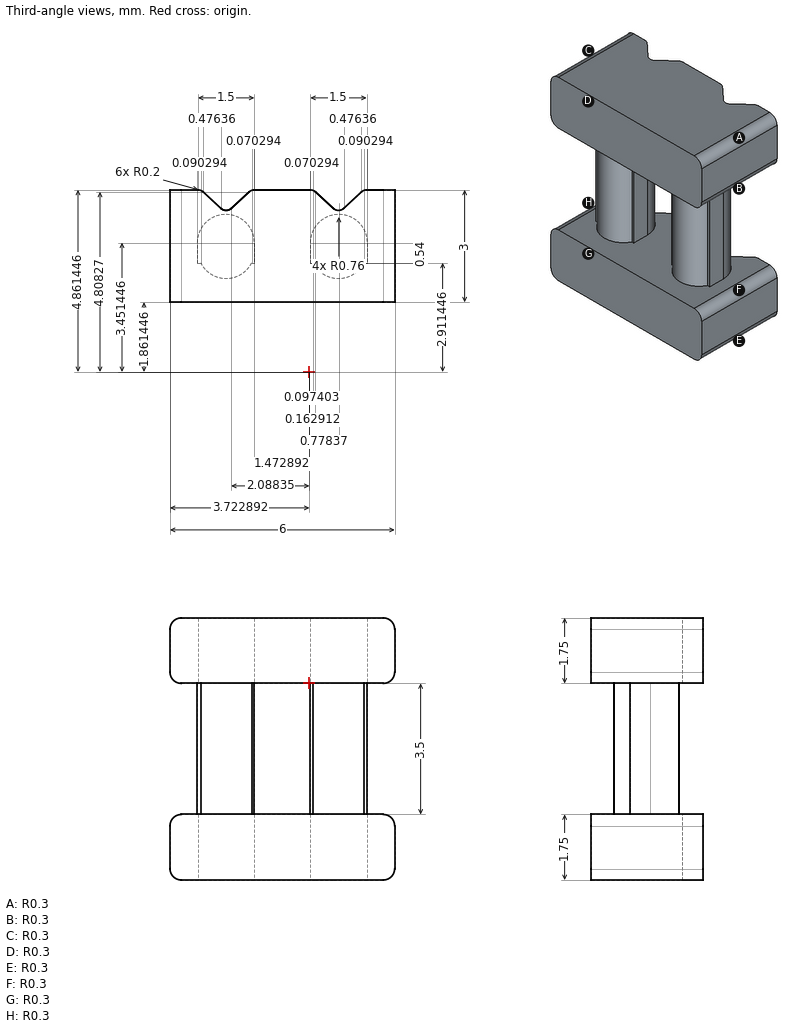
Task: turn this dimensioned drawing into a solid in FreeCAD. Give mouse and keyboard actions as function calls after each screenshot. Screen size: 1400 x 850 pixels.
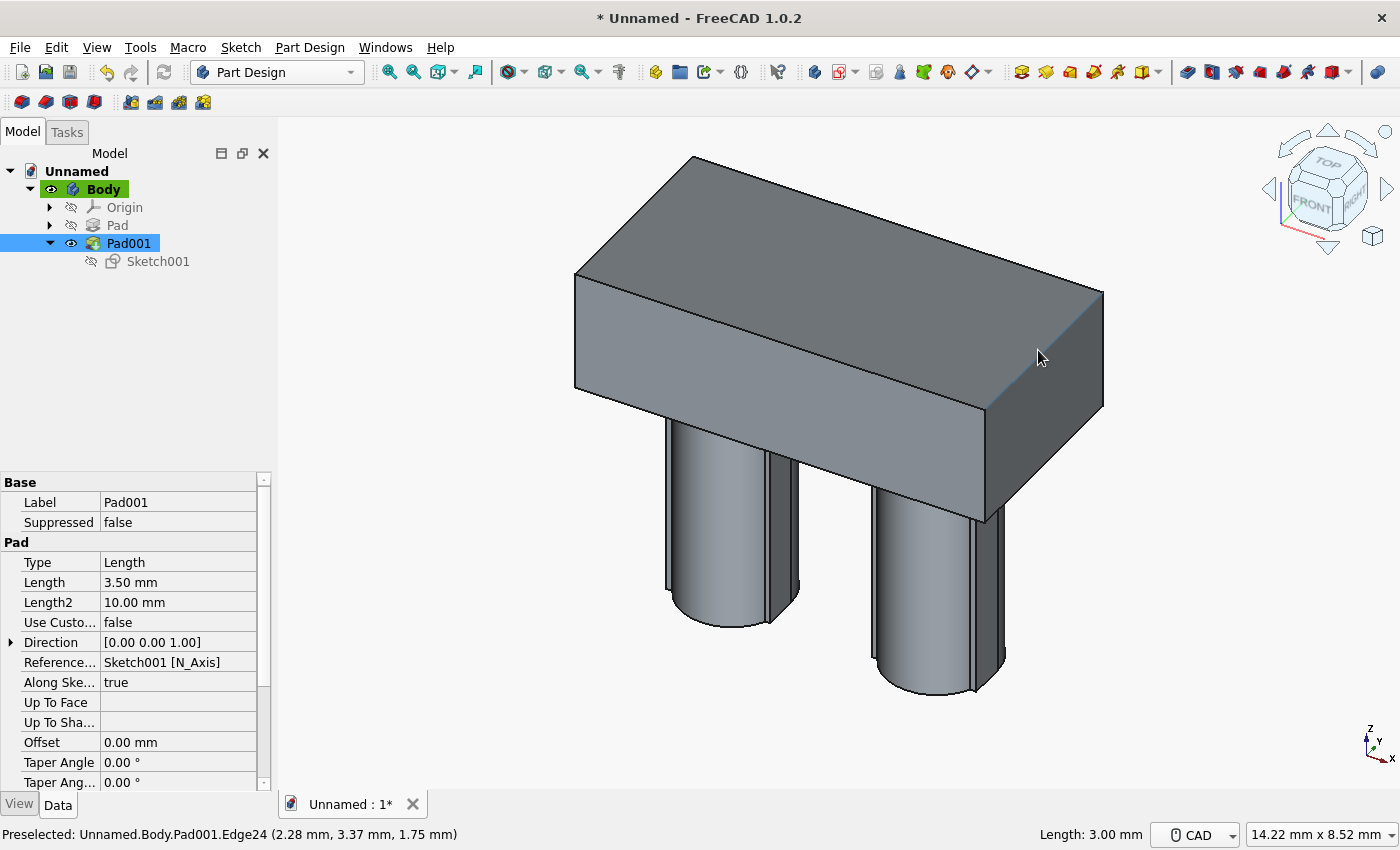
click(22, 102)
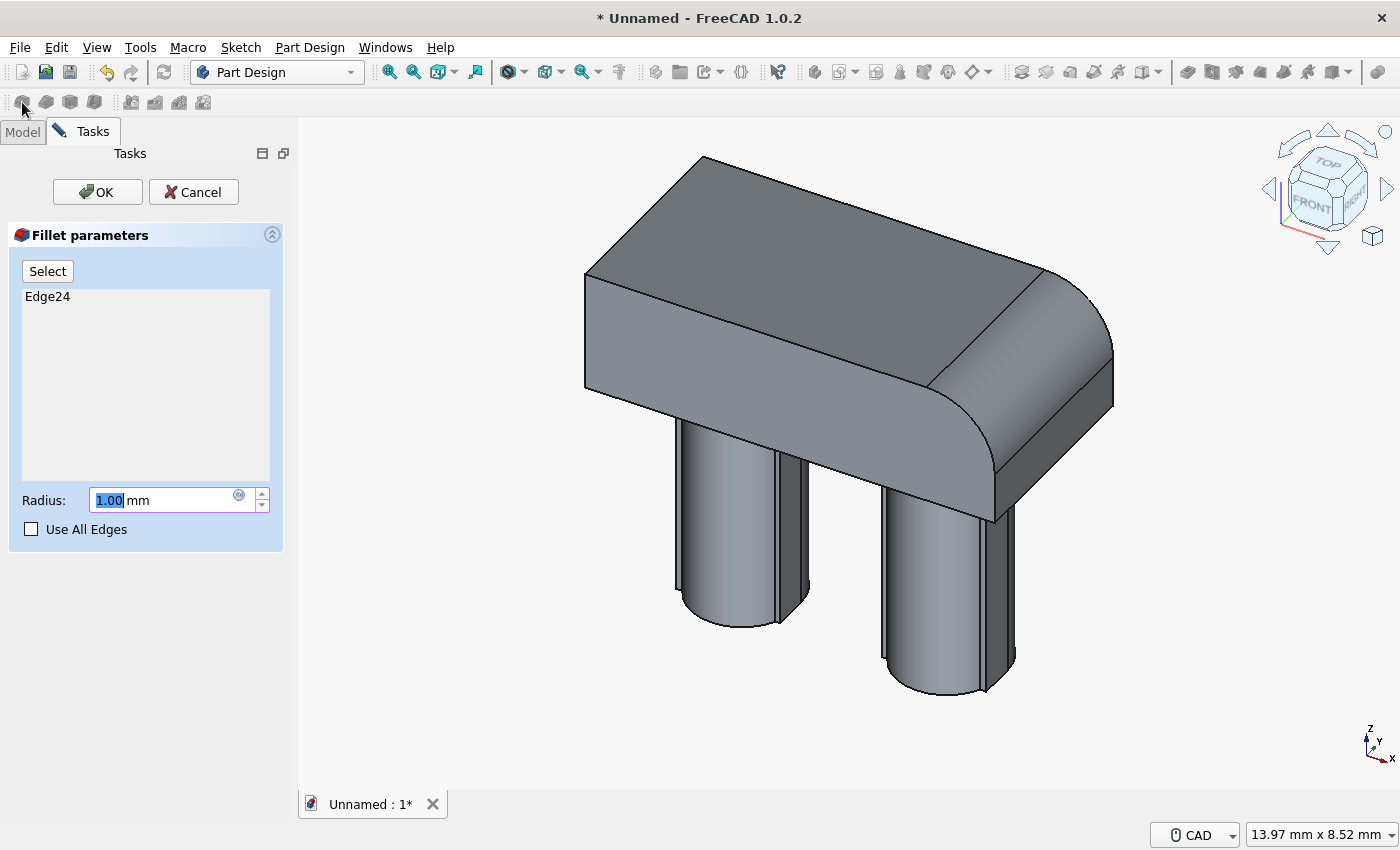
text(0.3)
key(Tab)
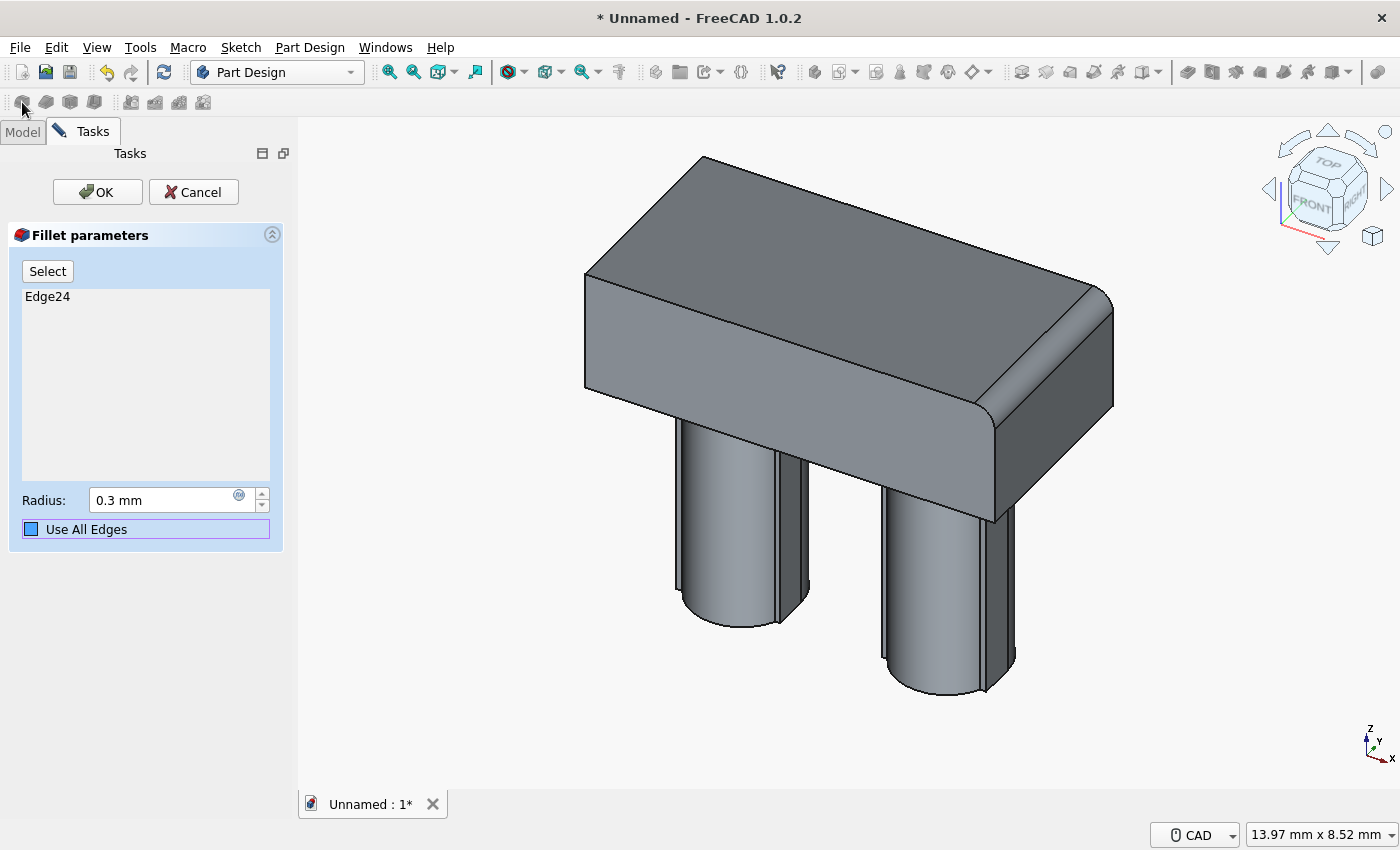
click(98, 192)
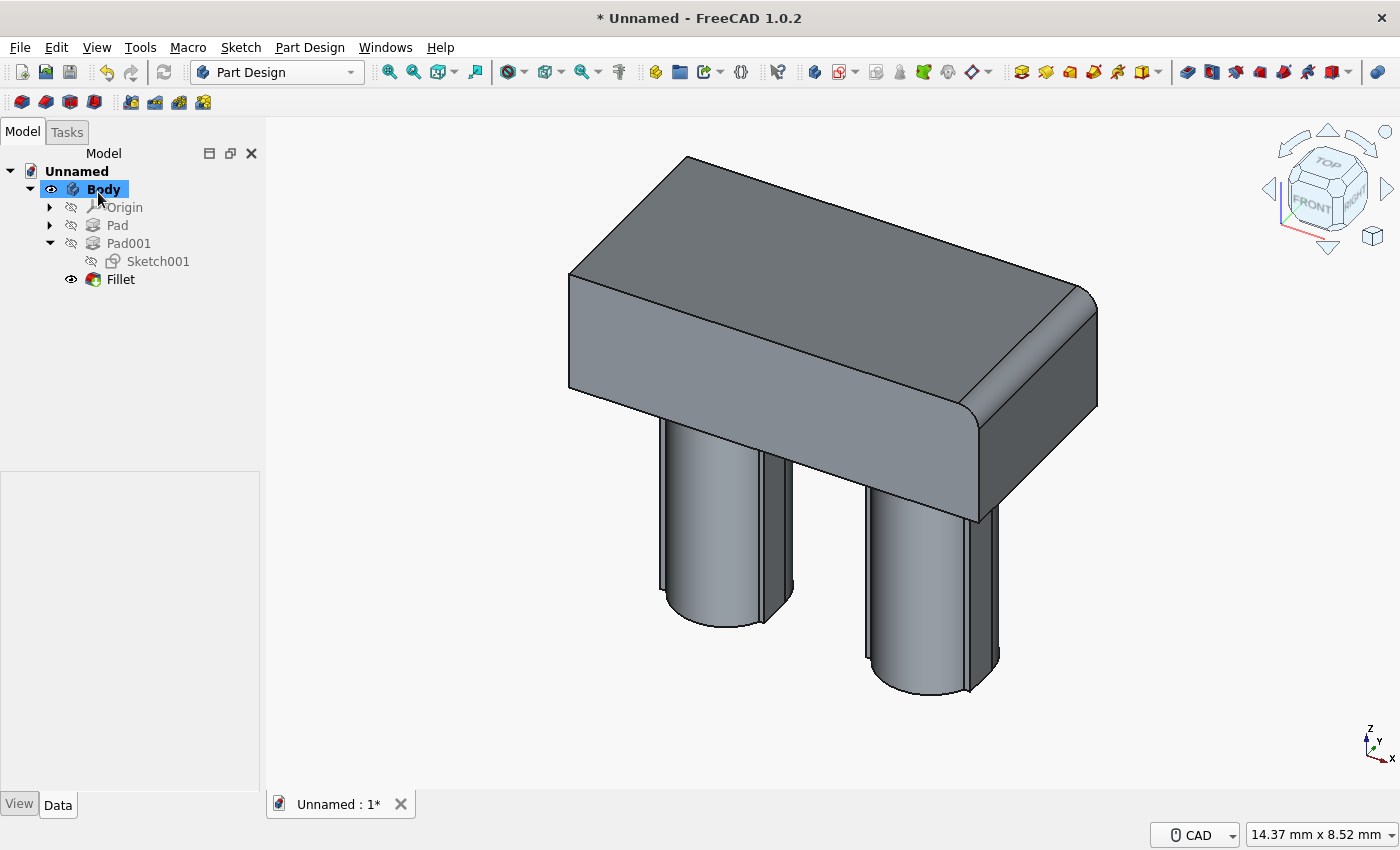
key(0)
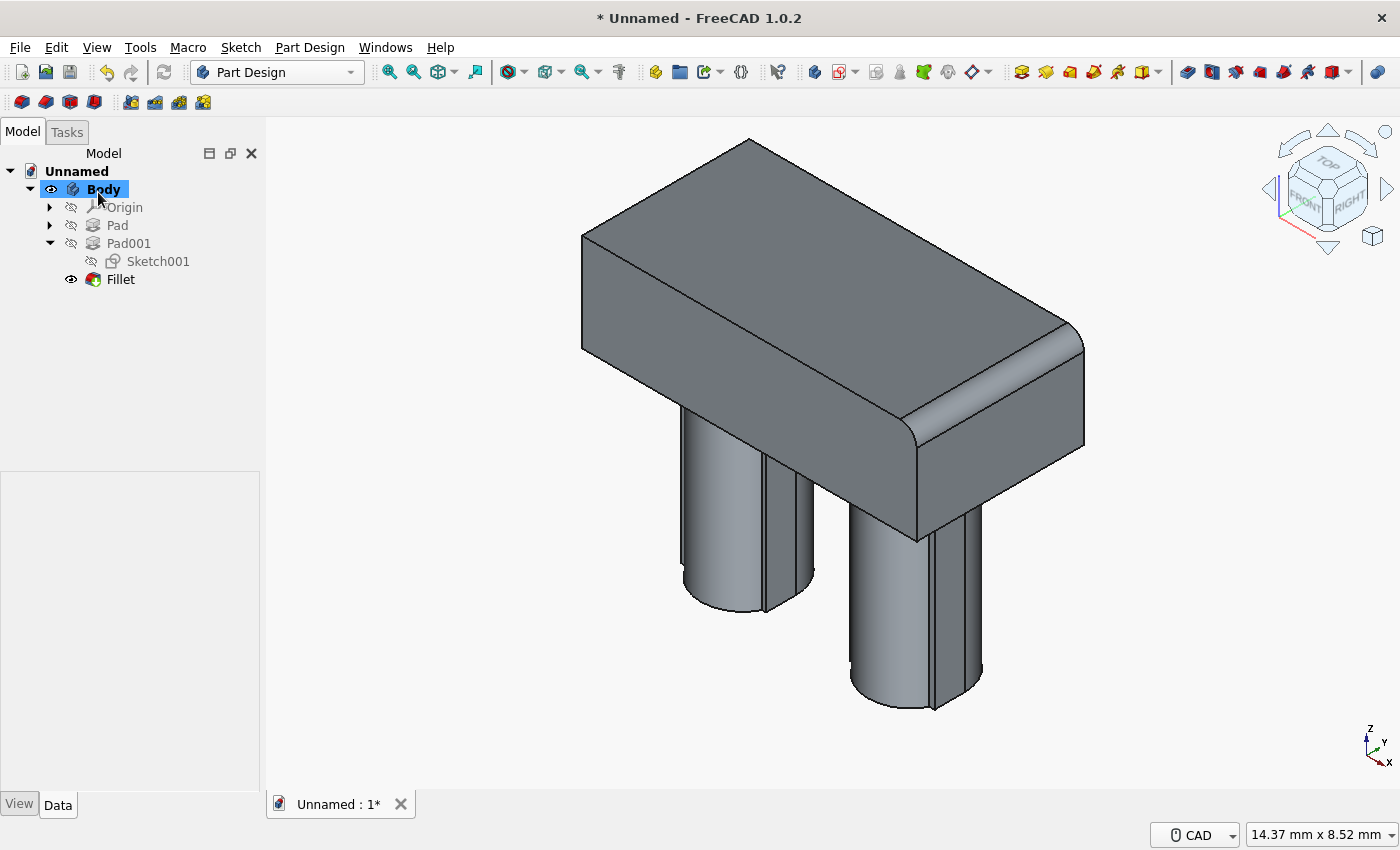
key(2)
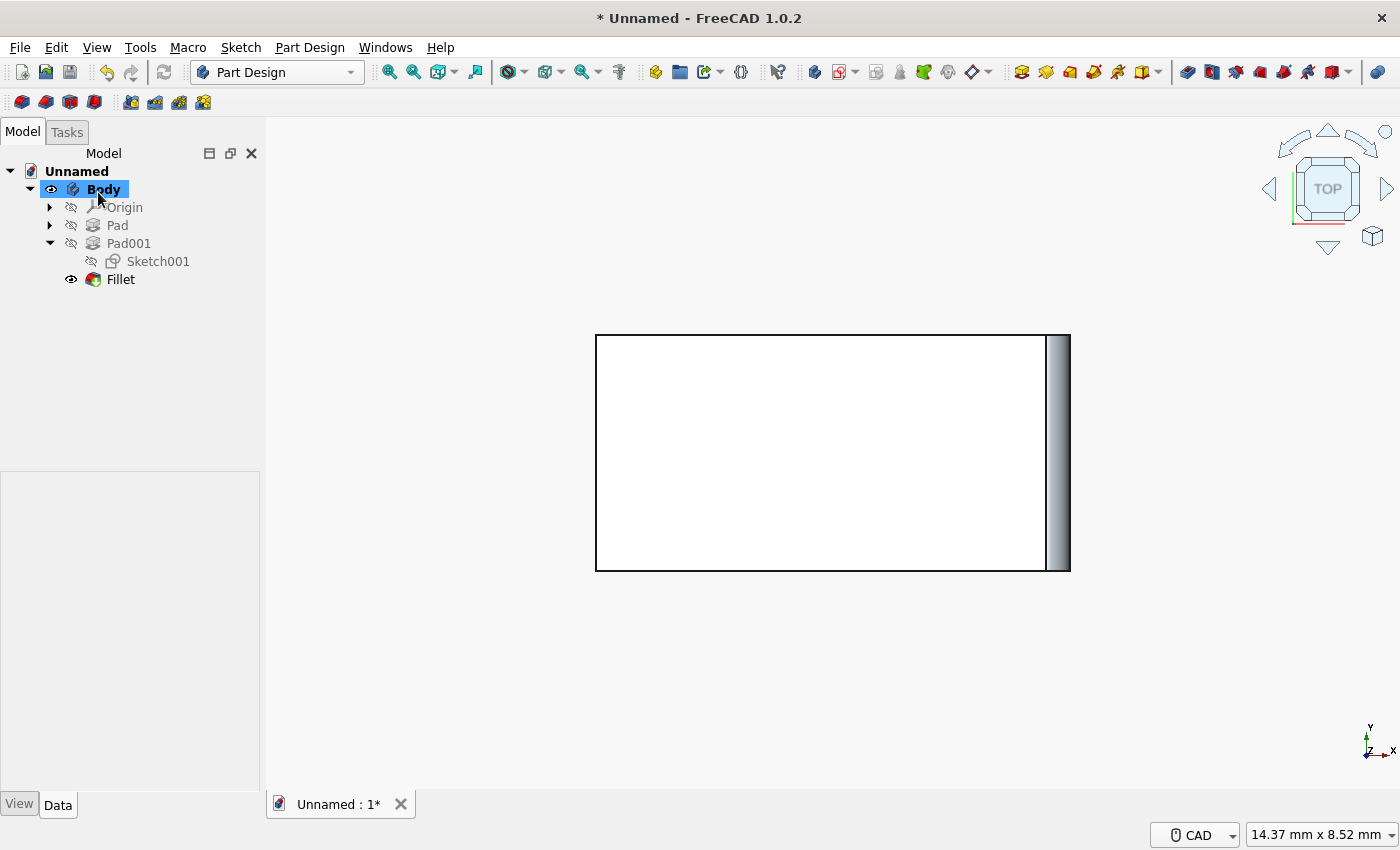
click(390, 72)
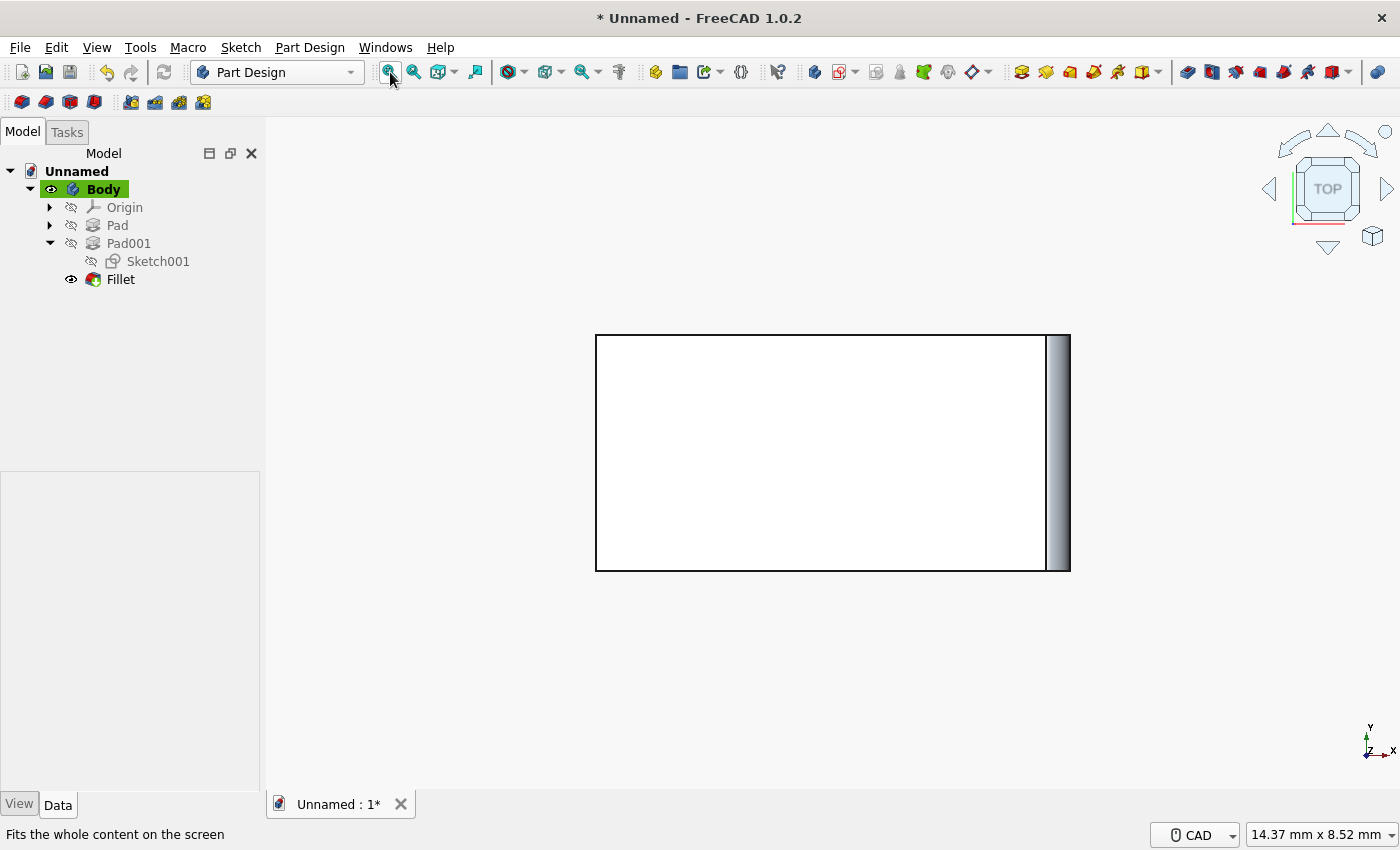
key(1)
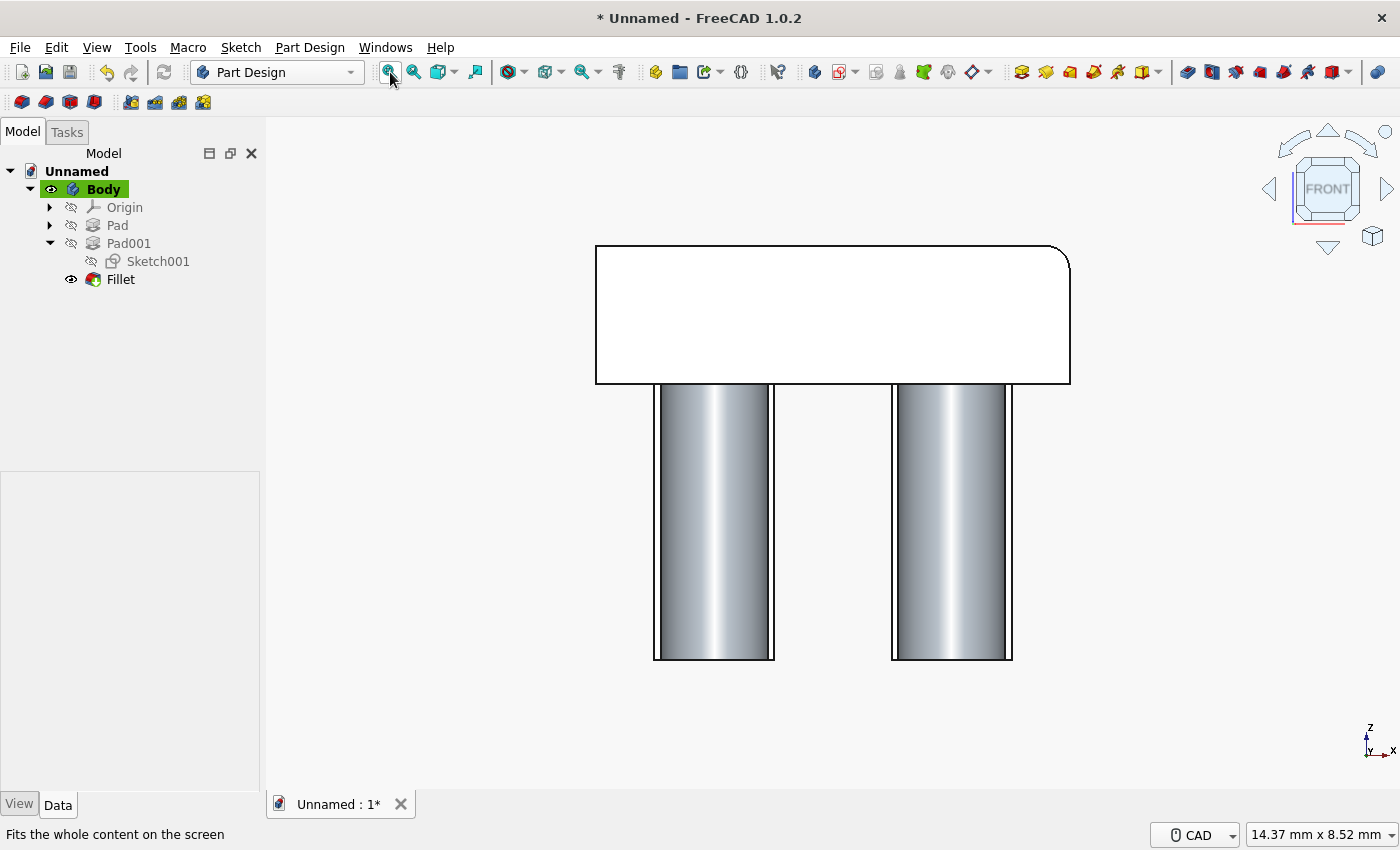
key(3)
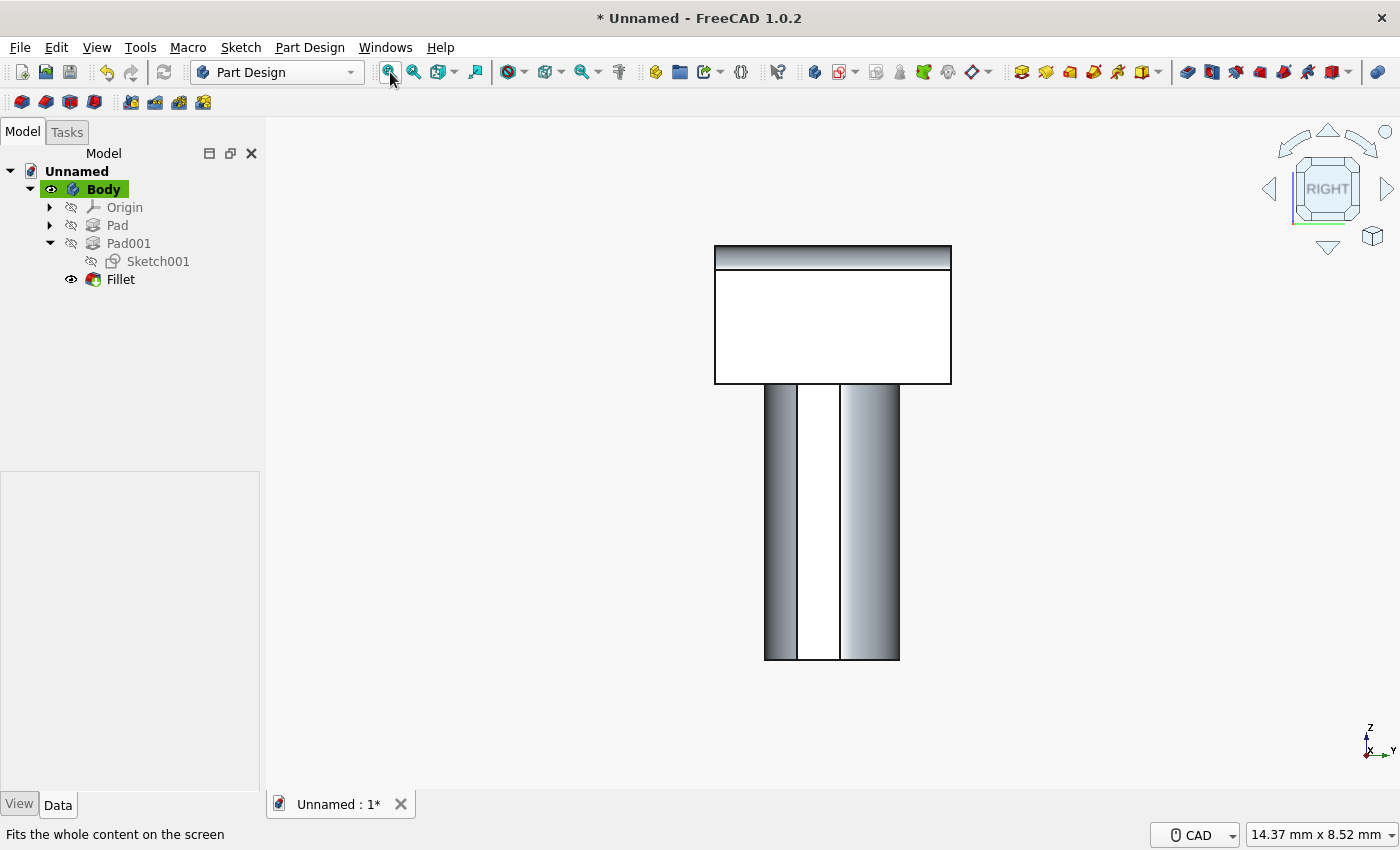
click(833, 383)